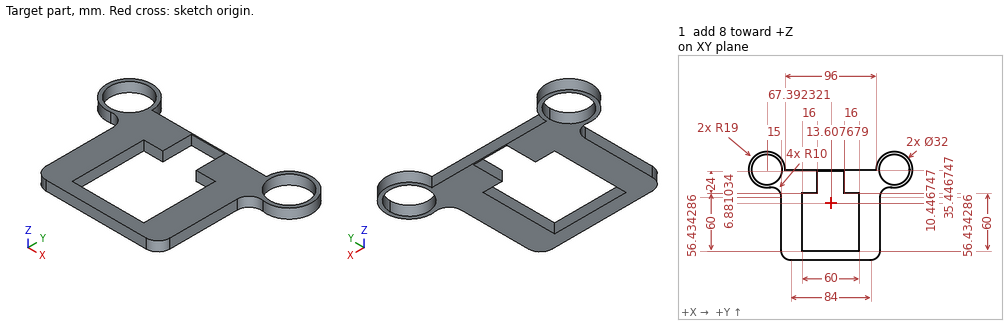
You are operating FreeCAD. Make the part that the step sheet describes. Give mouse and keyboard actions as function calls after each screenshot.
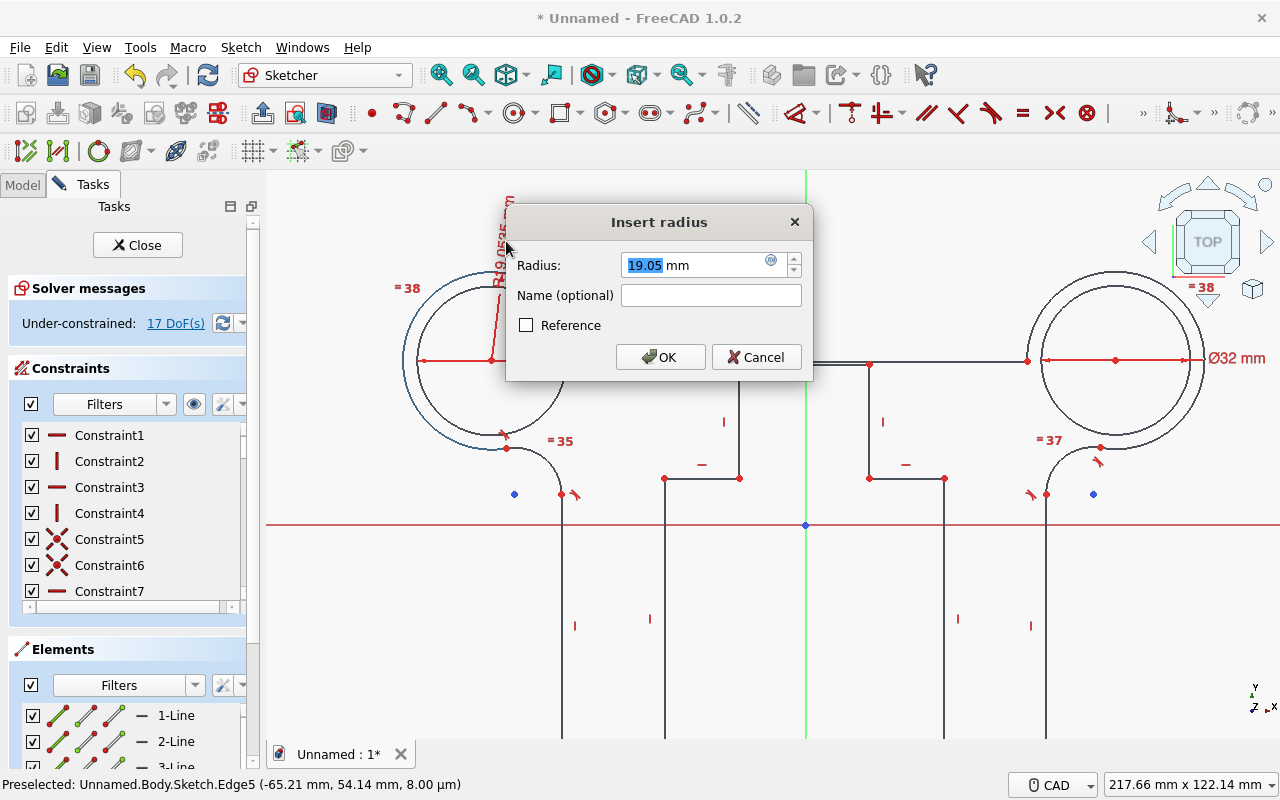
text(19)
key(Return)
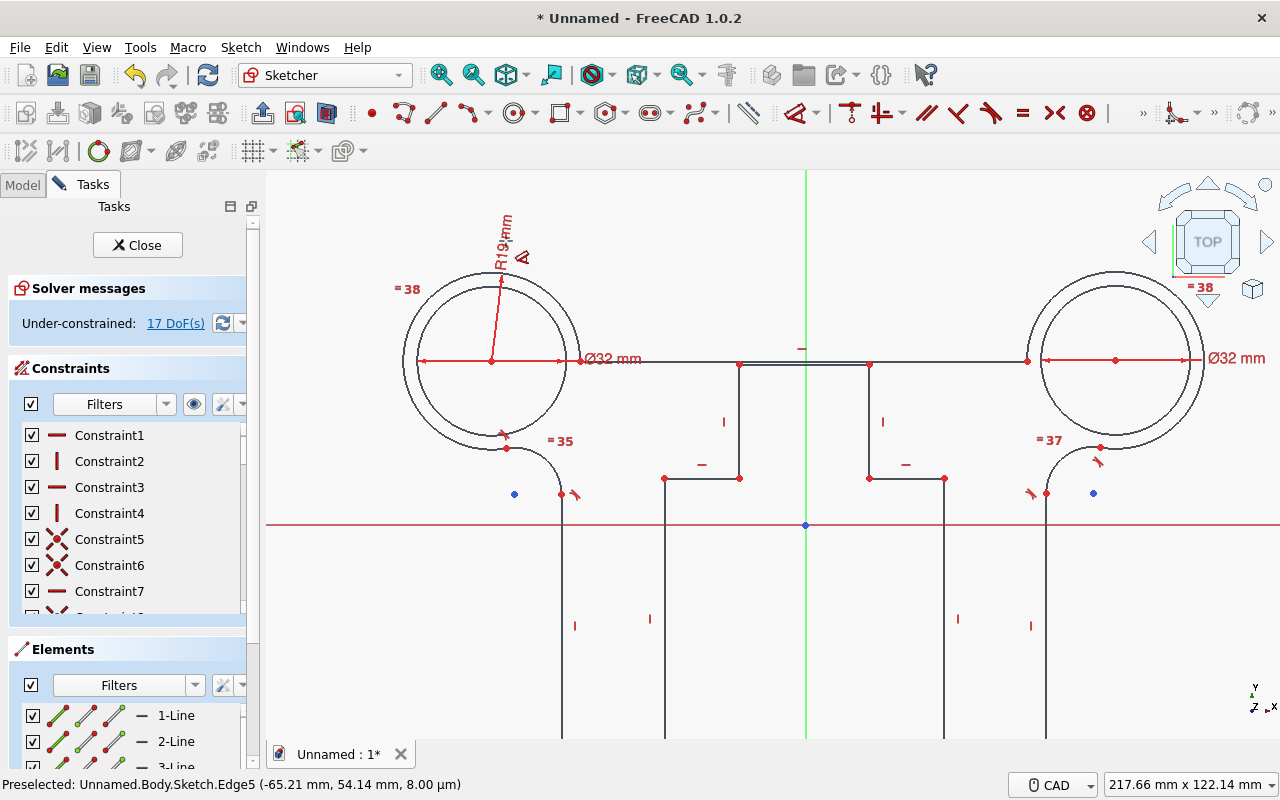
click(555, 471)
click(583, 455)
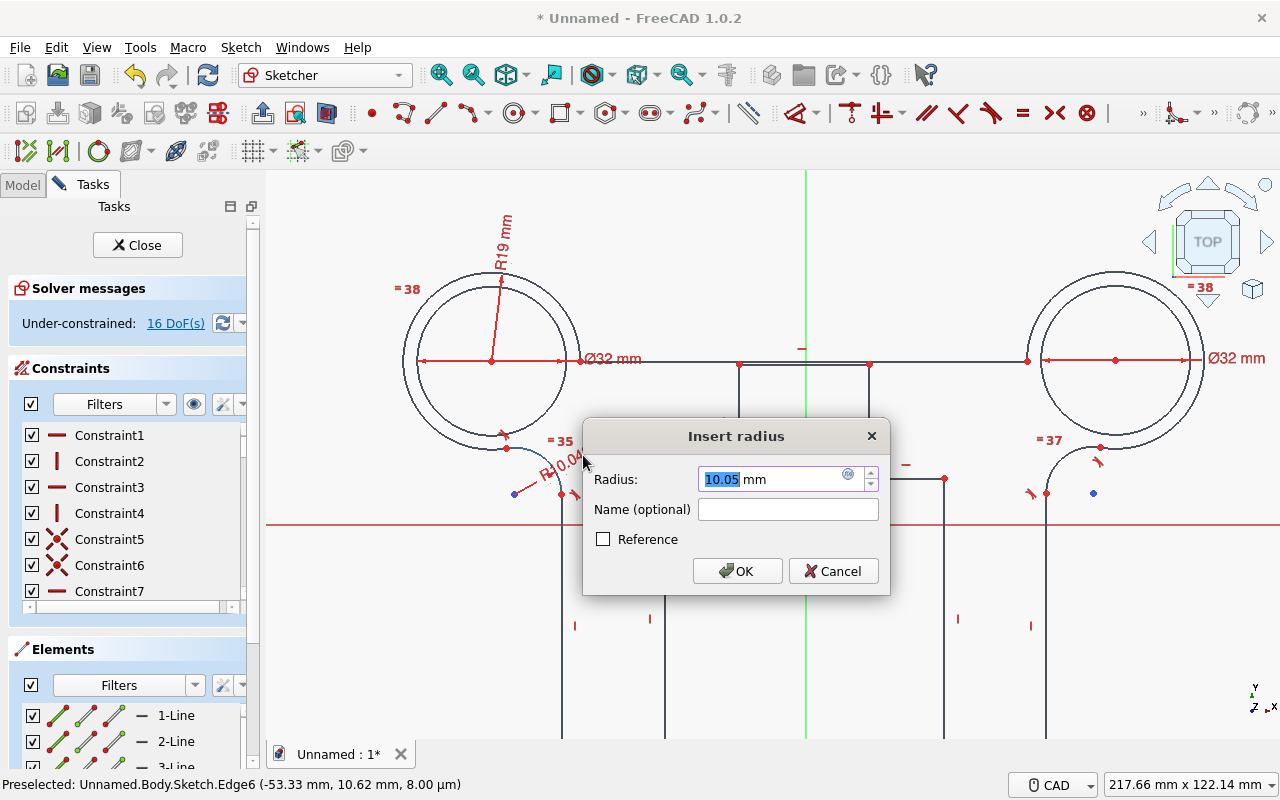
text(10)
key(Return)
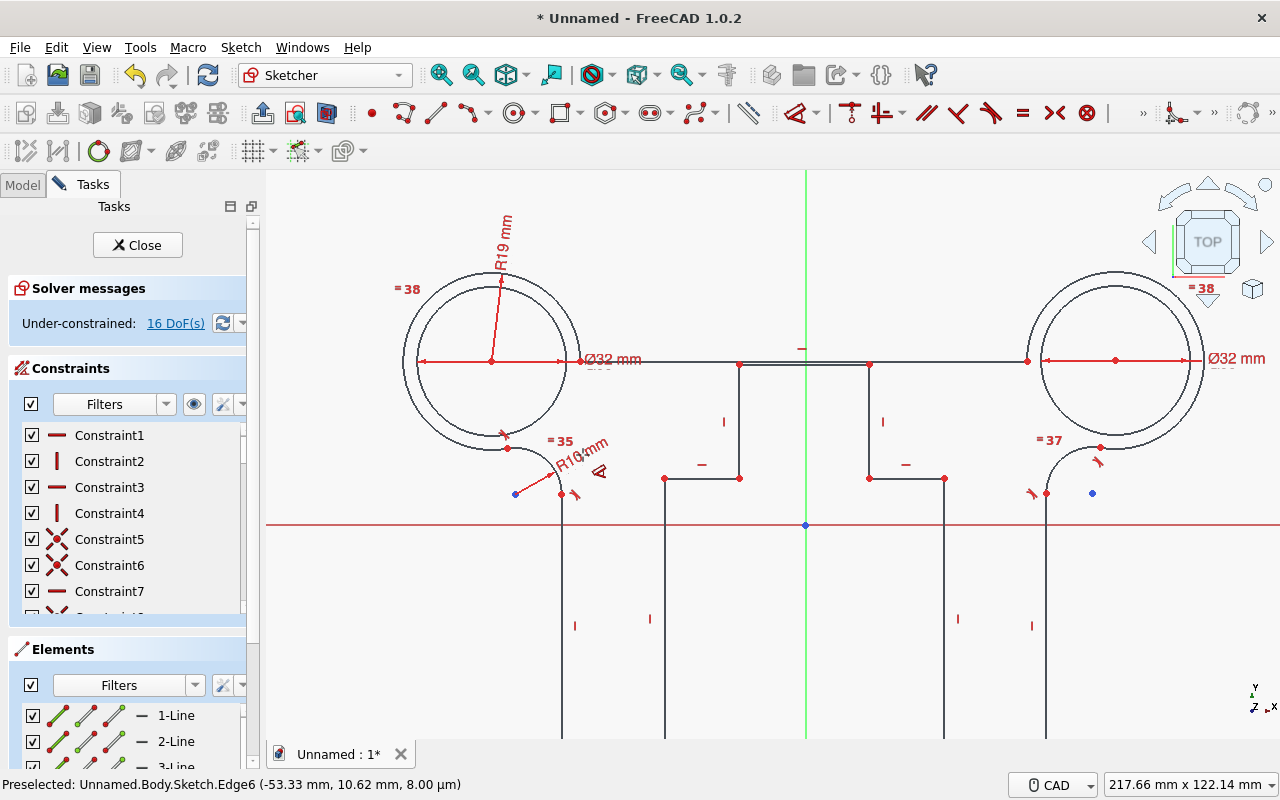
click(893, 362)
click(701, 328)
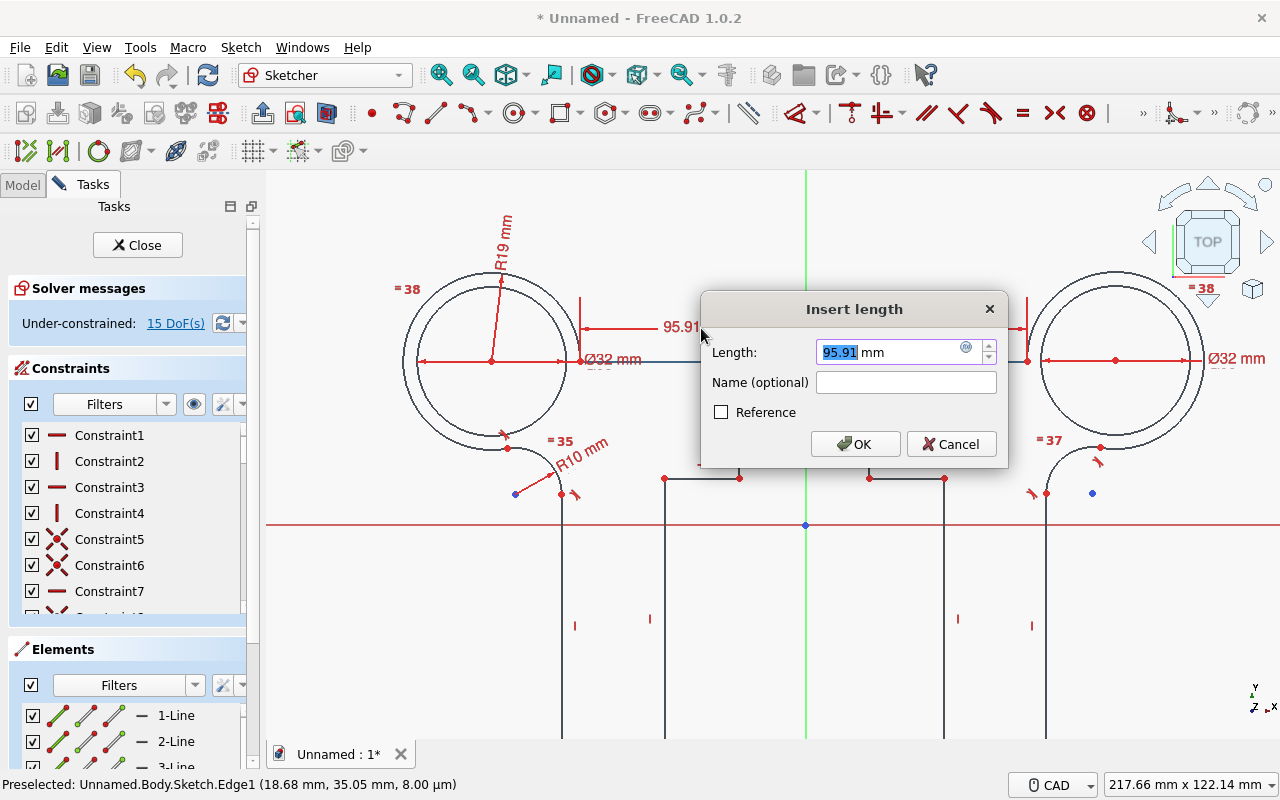
text(96)
key(Return)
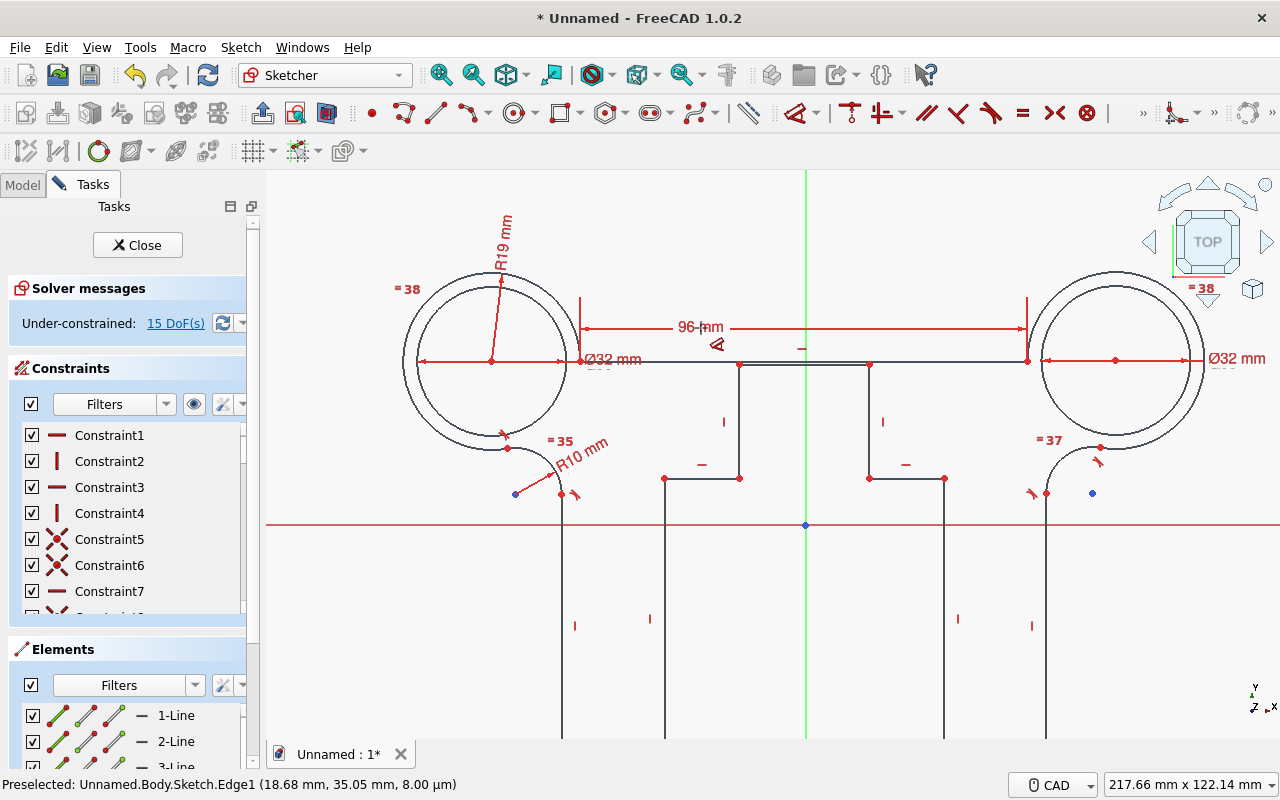
scroll(502, 273, down, 2)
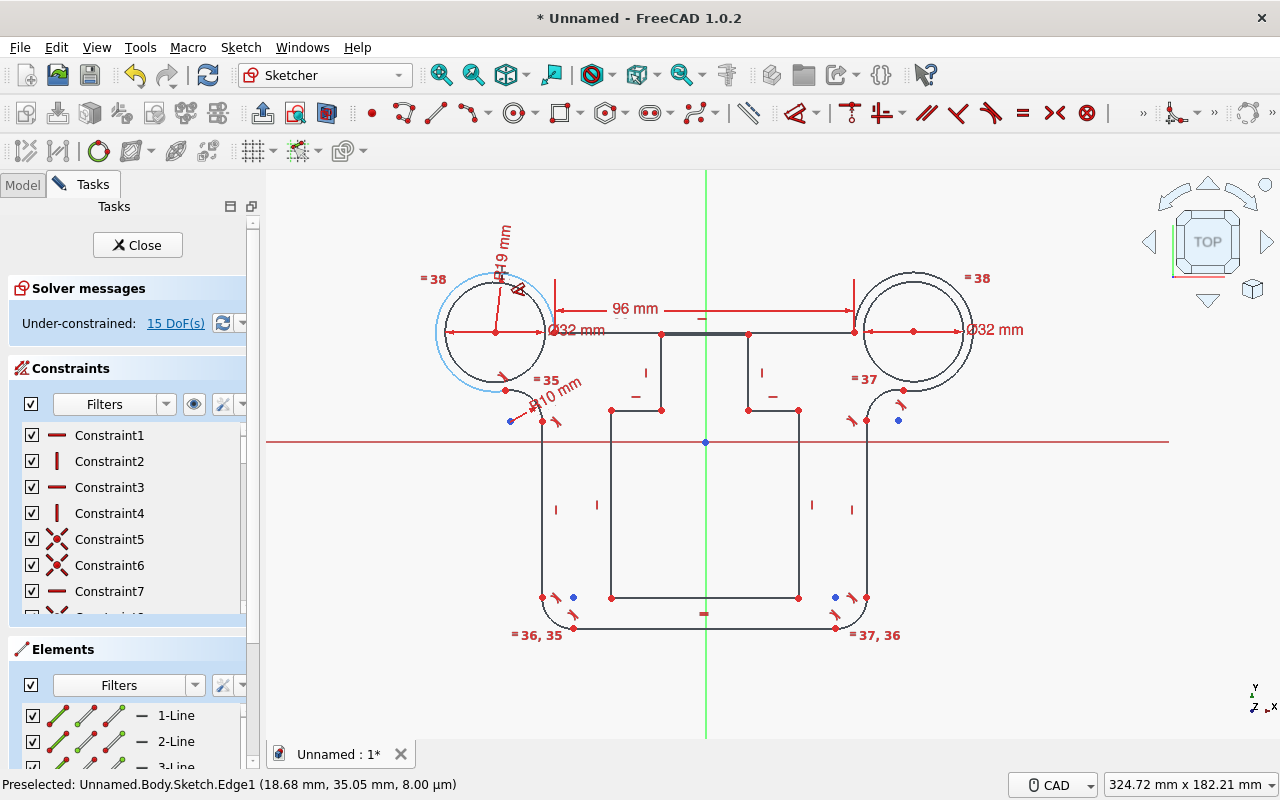
click(652, 629)
click(644, 663)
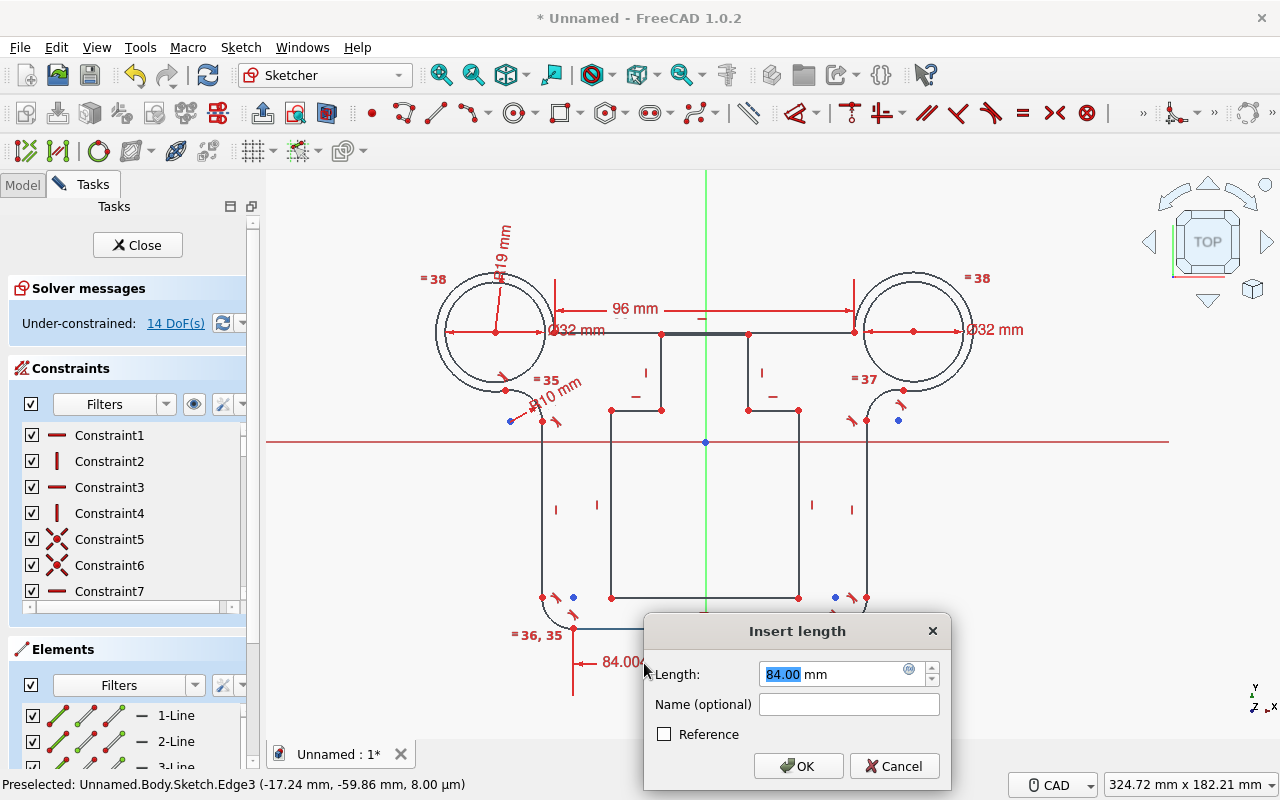
text(84)
key(Return)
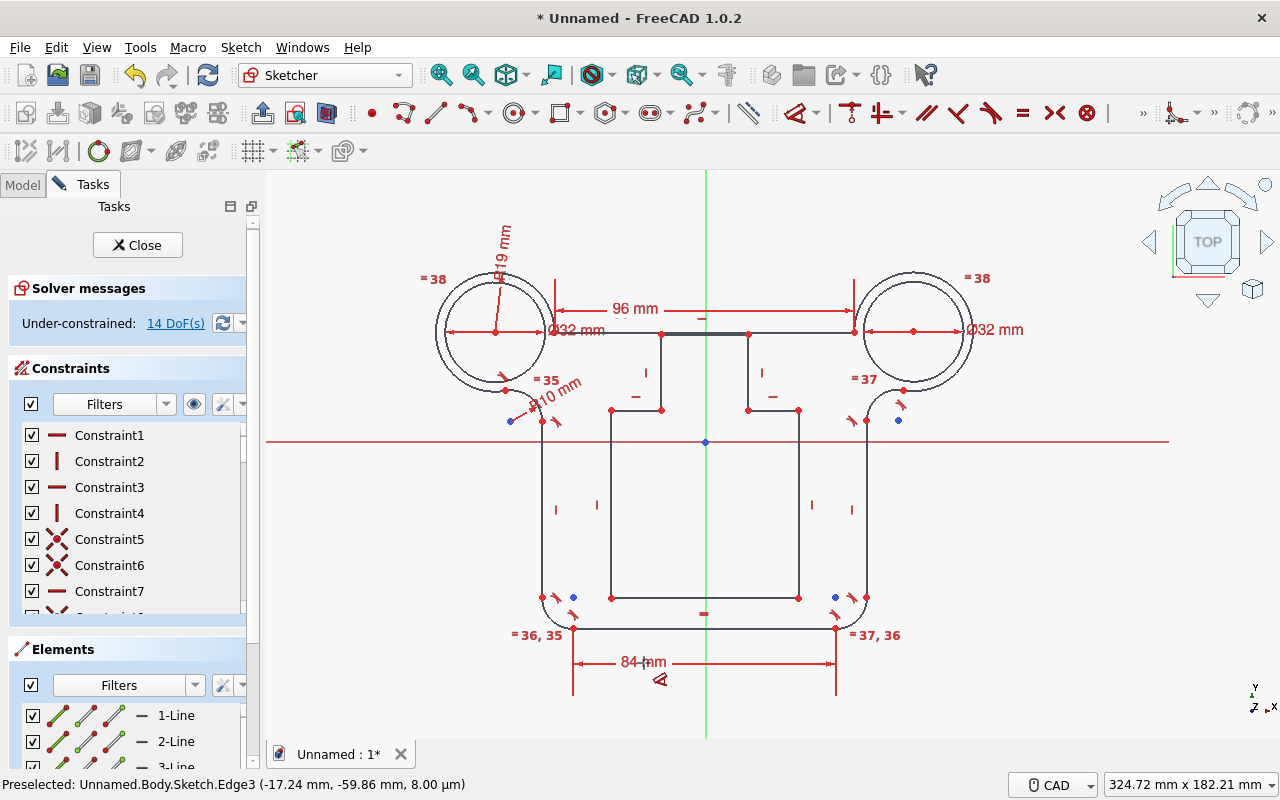
click(763, 411)
click(773, 377)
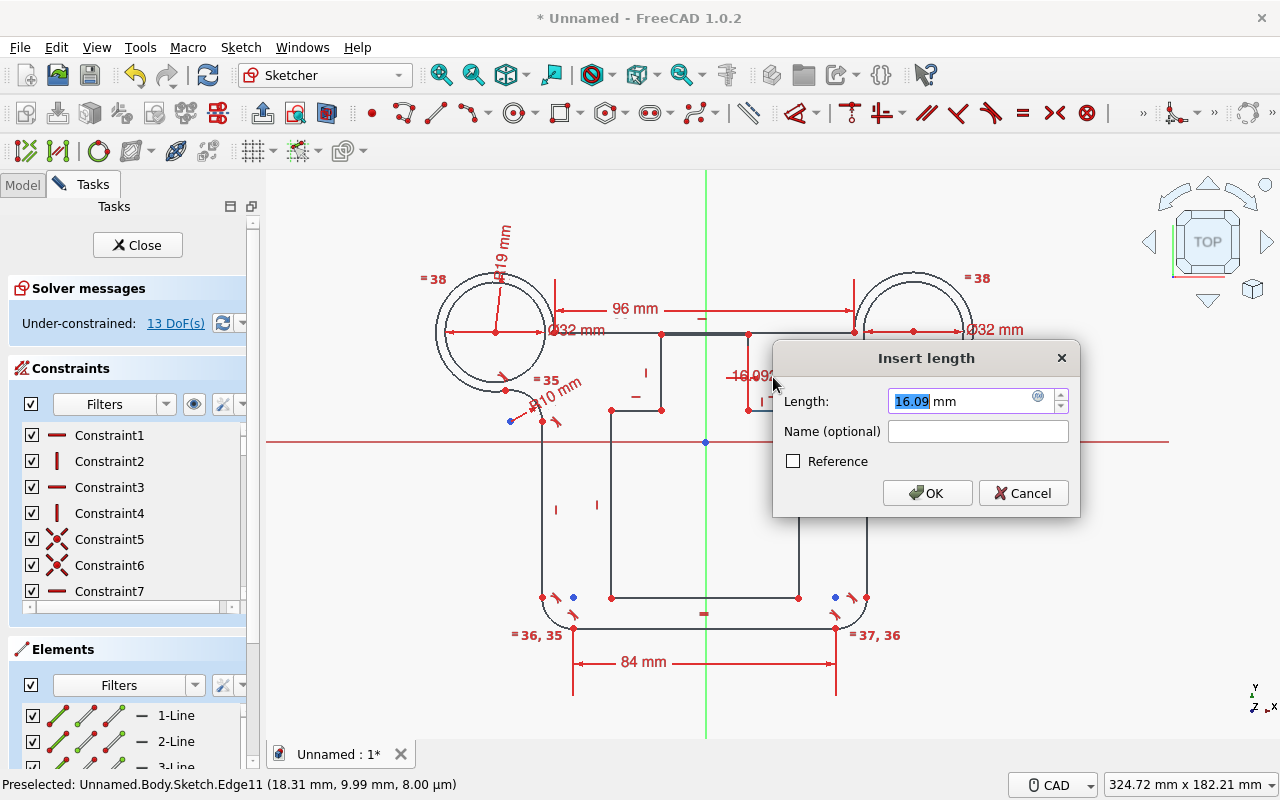
text(16)
key(Return)